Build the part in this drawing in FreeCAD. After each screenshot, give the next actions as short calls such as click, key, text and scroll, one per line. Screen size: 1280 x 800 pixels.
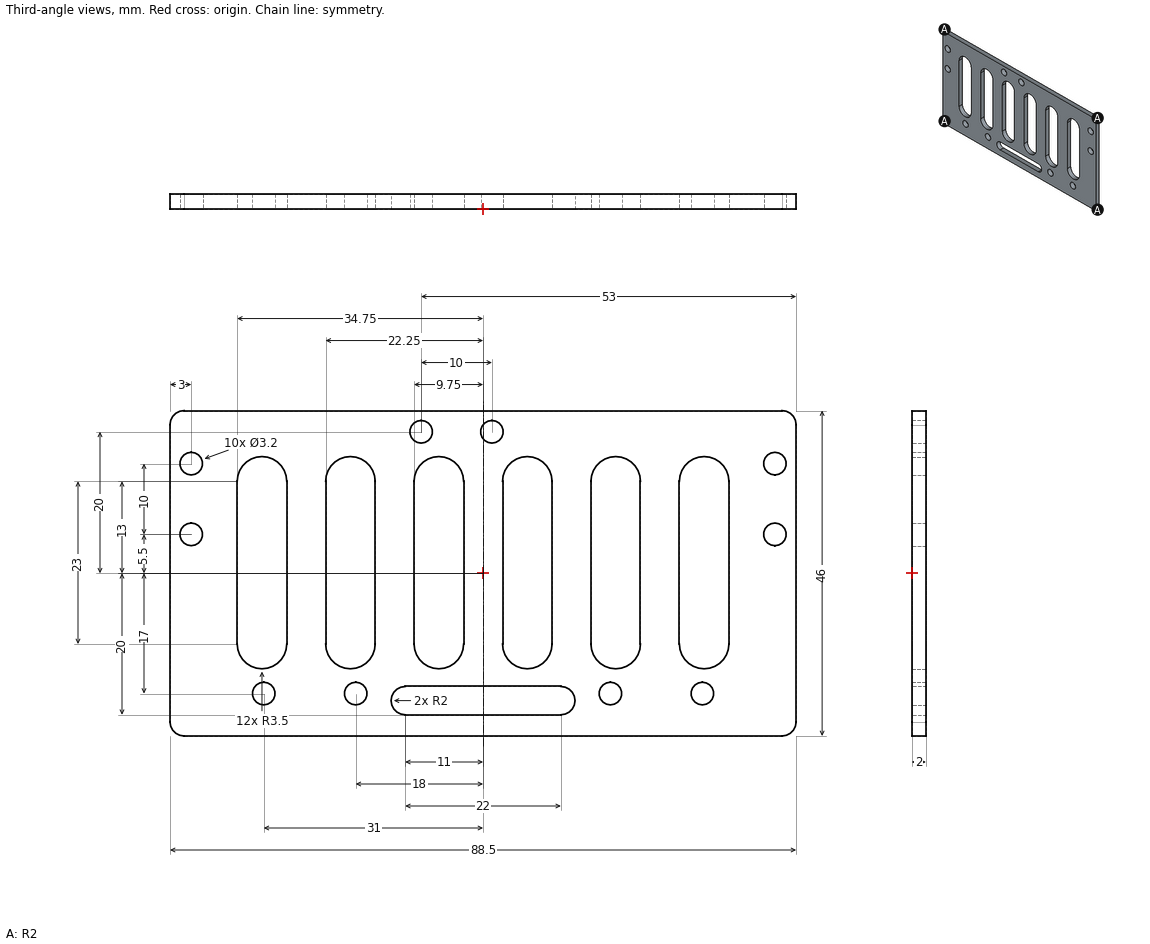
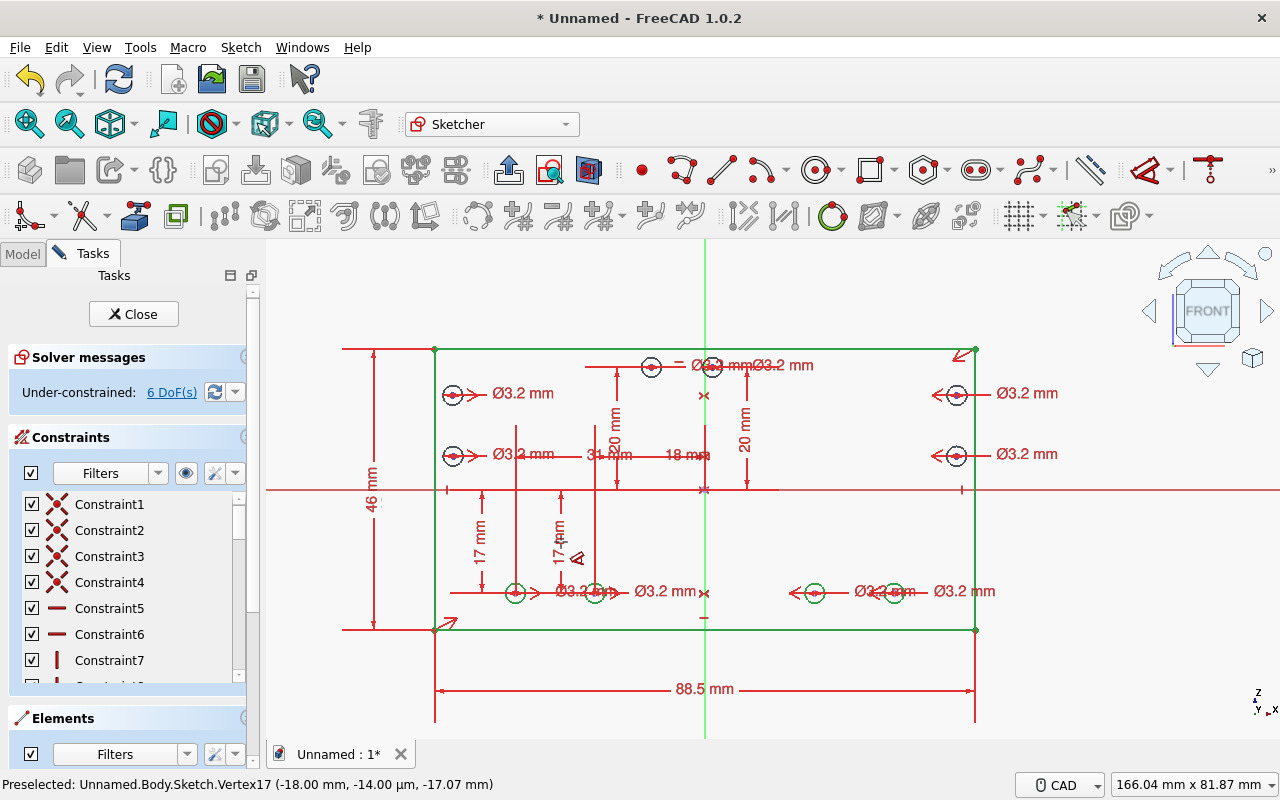
scroll(435, 349, up, 4)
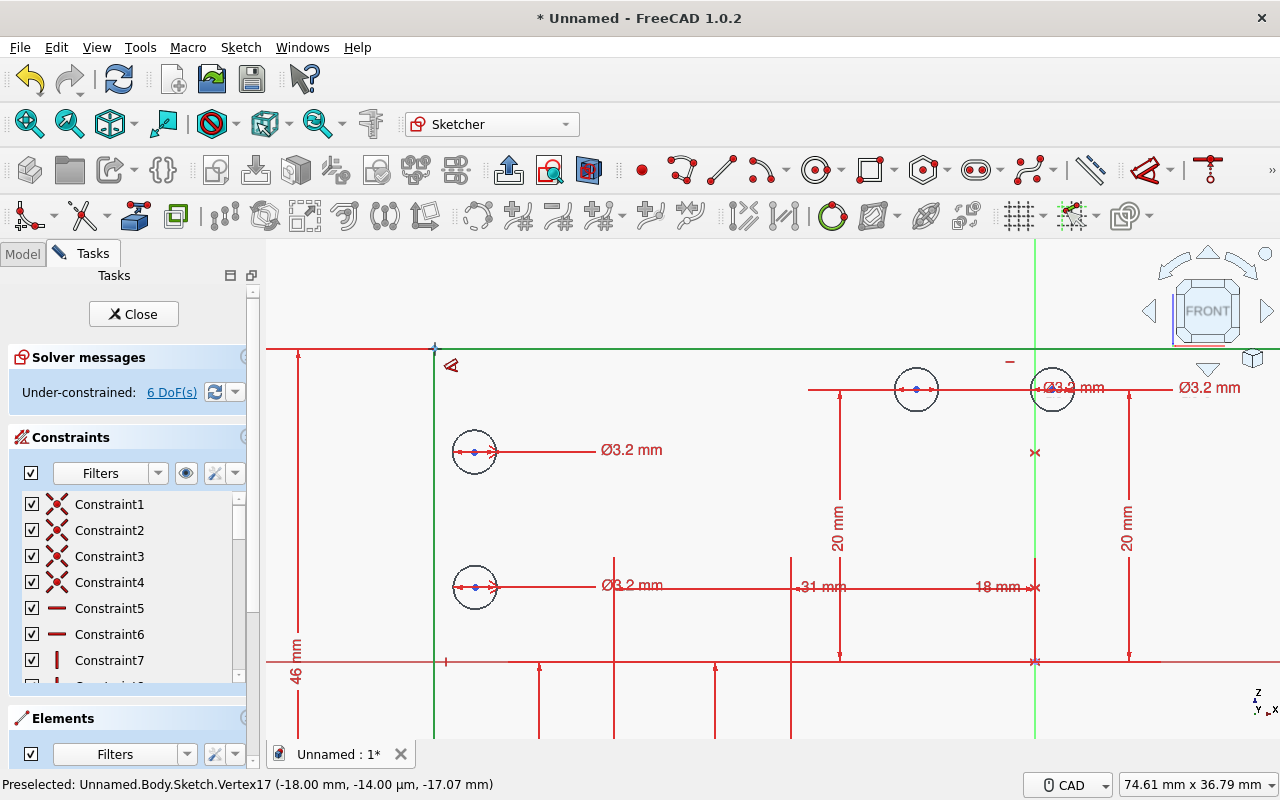
click(434, 349)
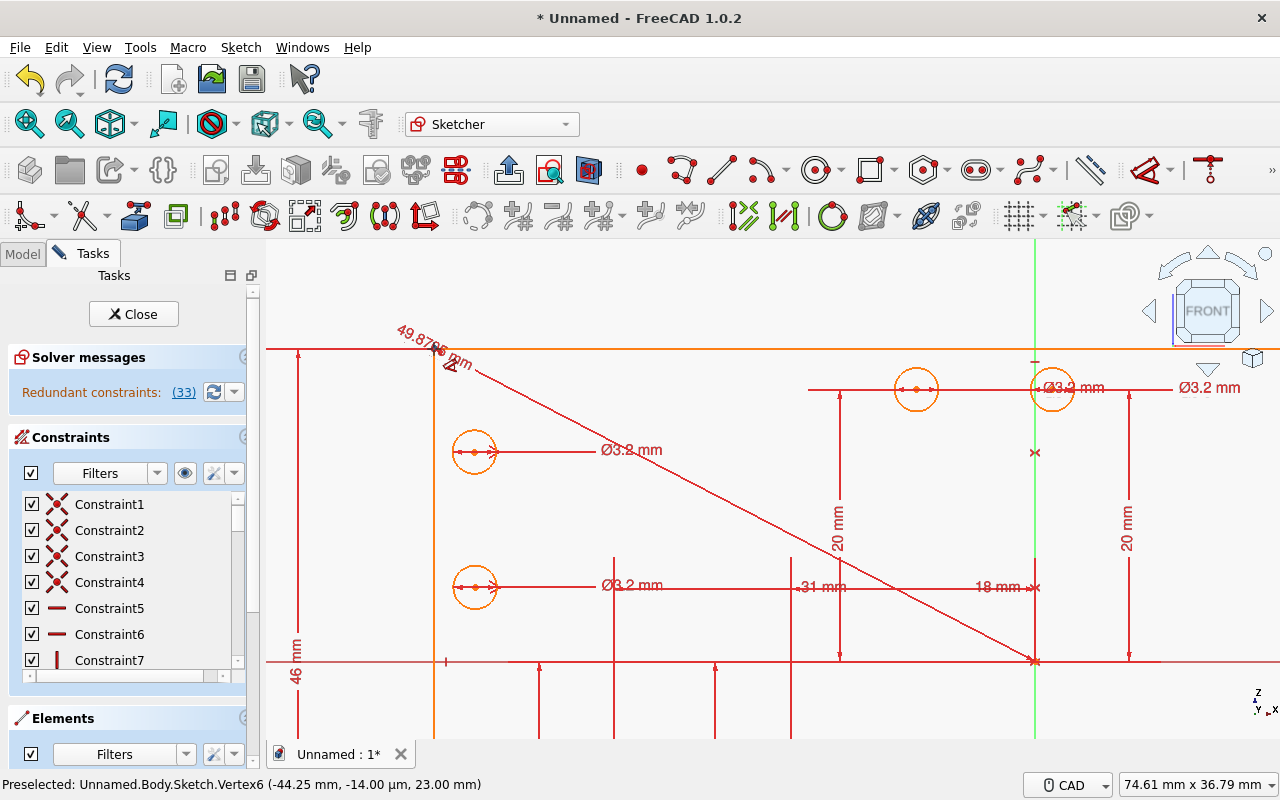
click(474, 452)
click(454, 315)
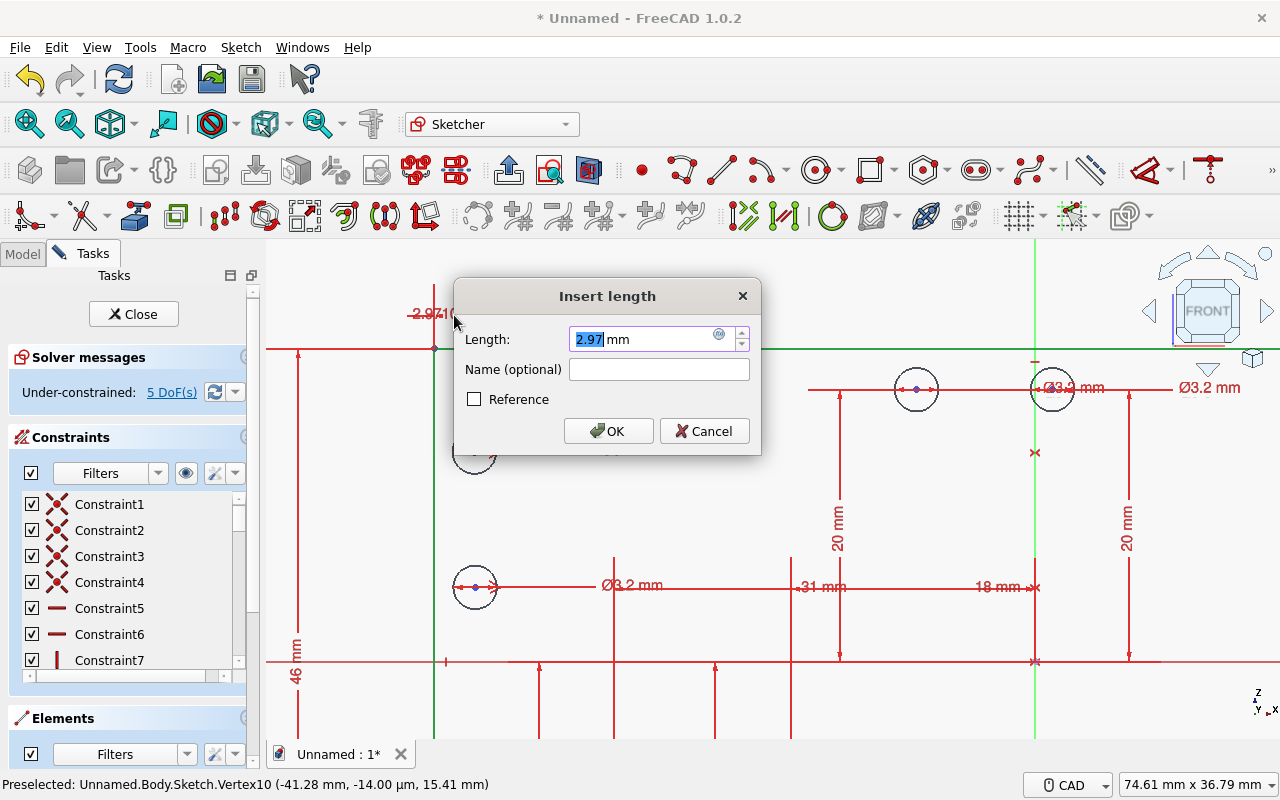
text(3)
key(Return)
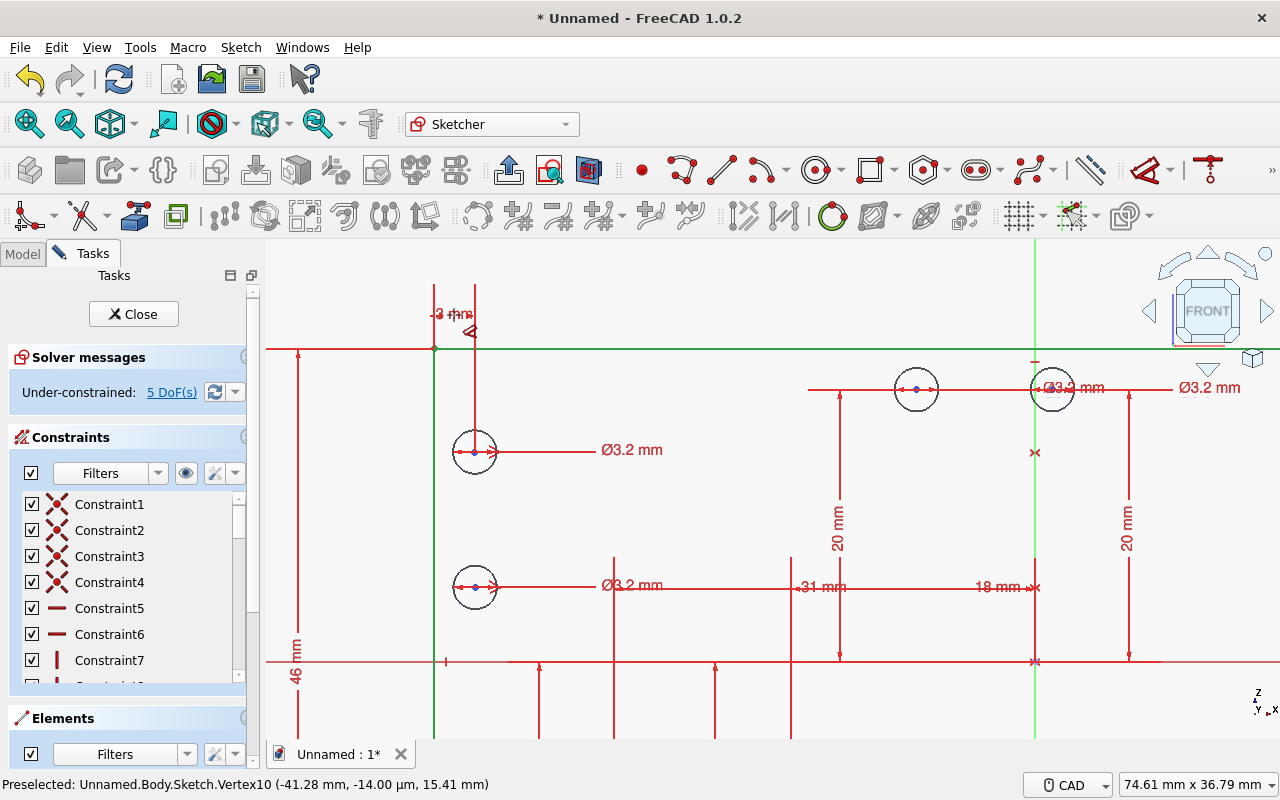
click(434, 349)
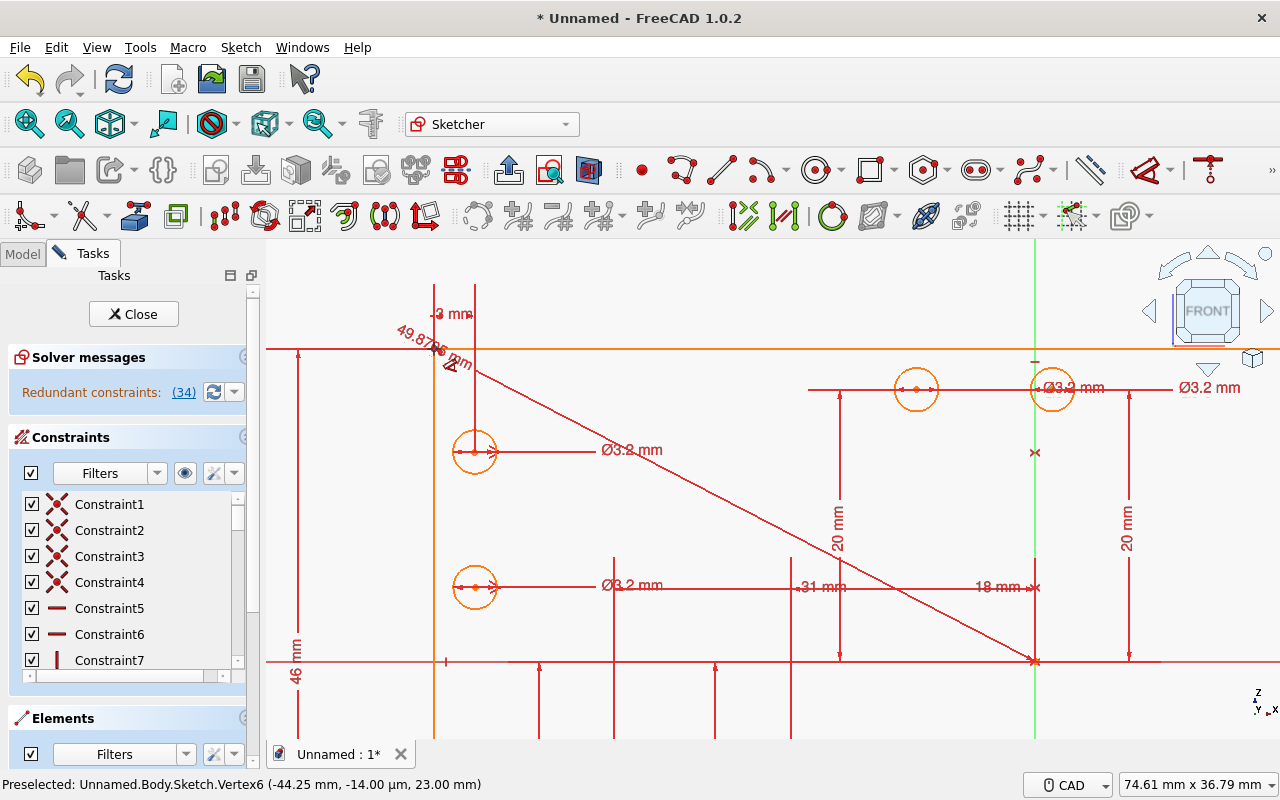
click(475, 587)
click(455, 621)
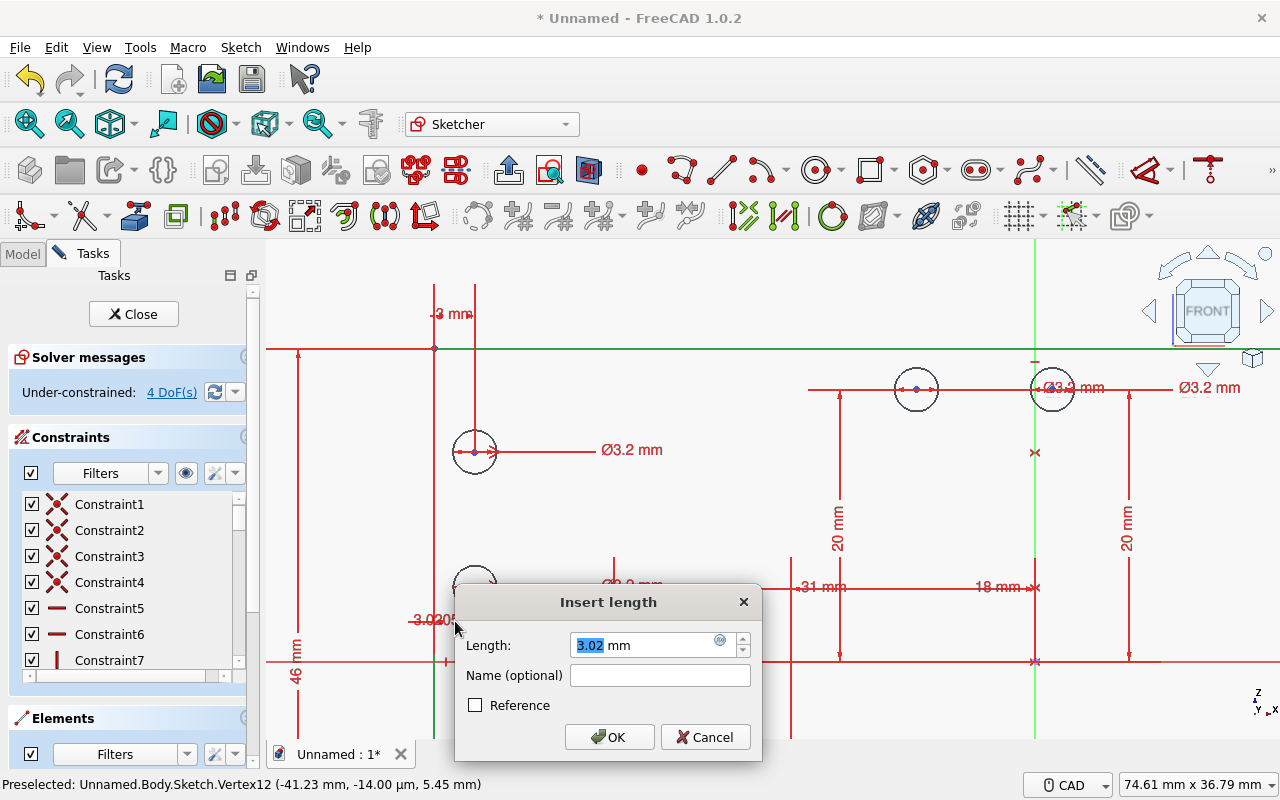
text(3)
key(Return)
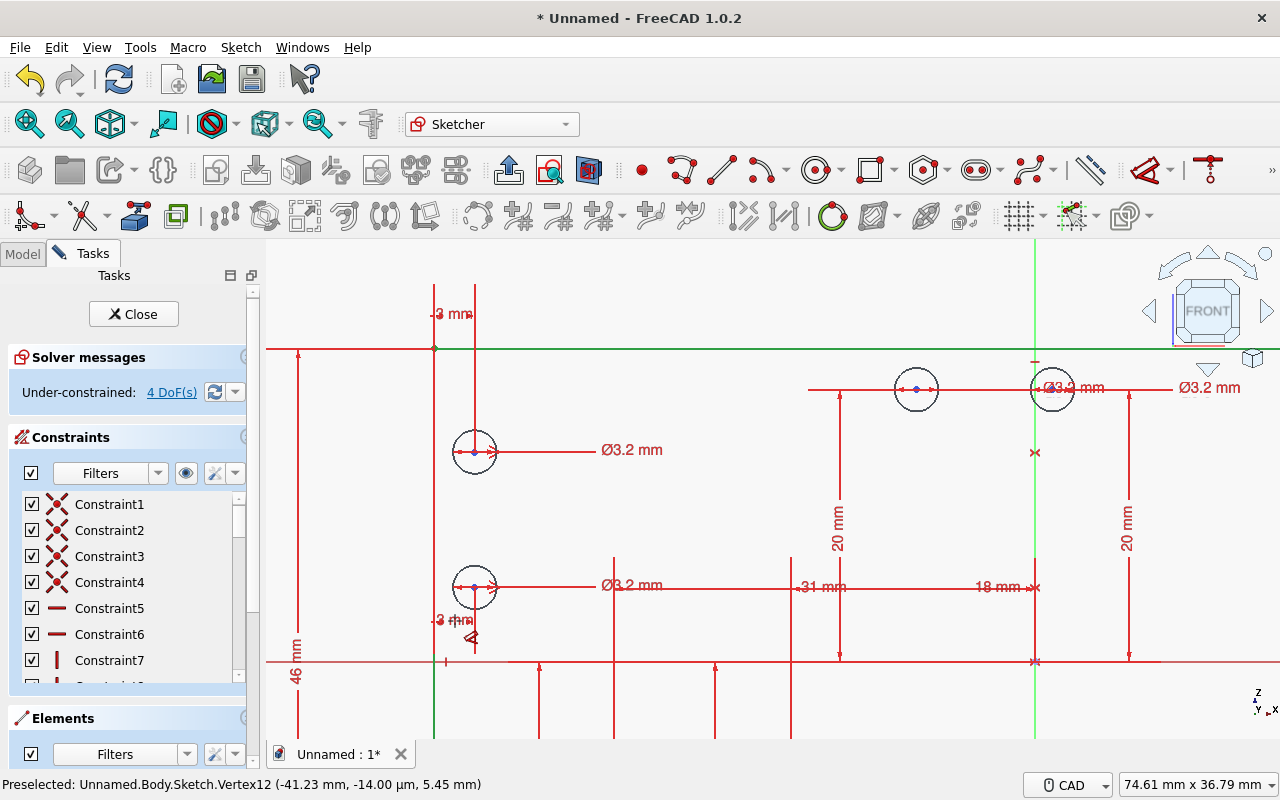
click(475, 587)
click(1069, 624)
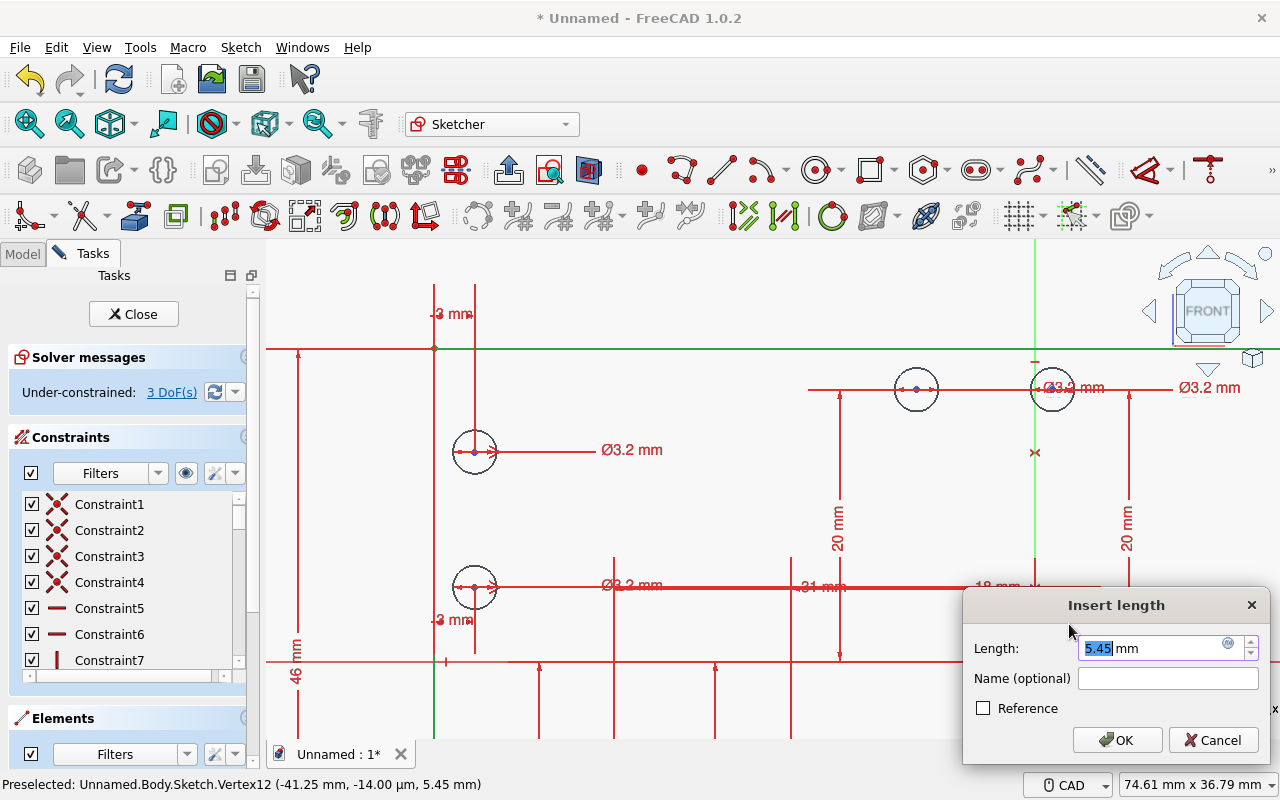
text(5.5)
key(Return)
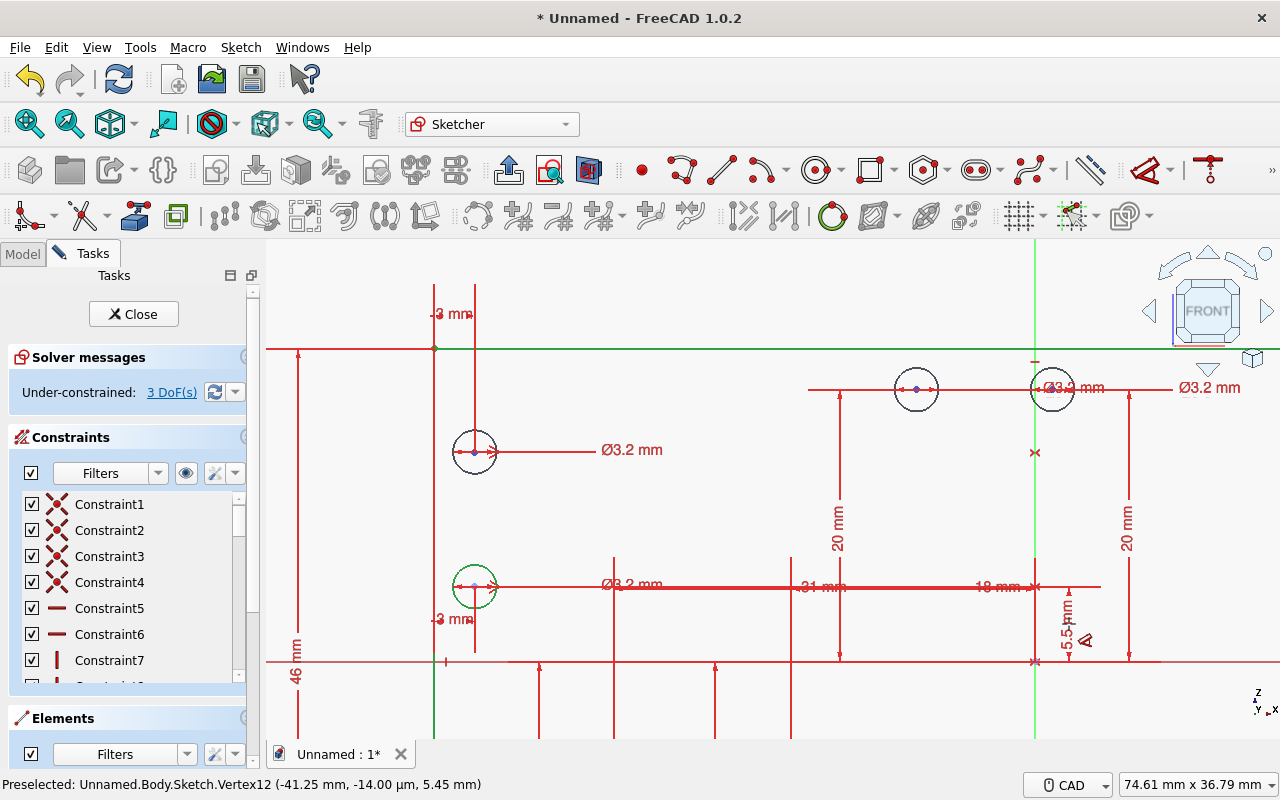
scroll(434, 348, down, 4)